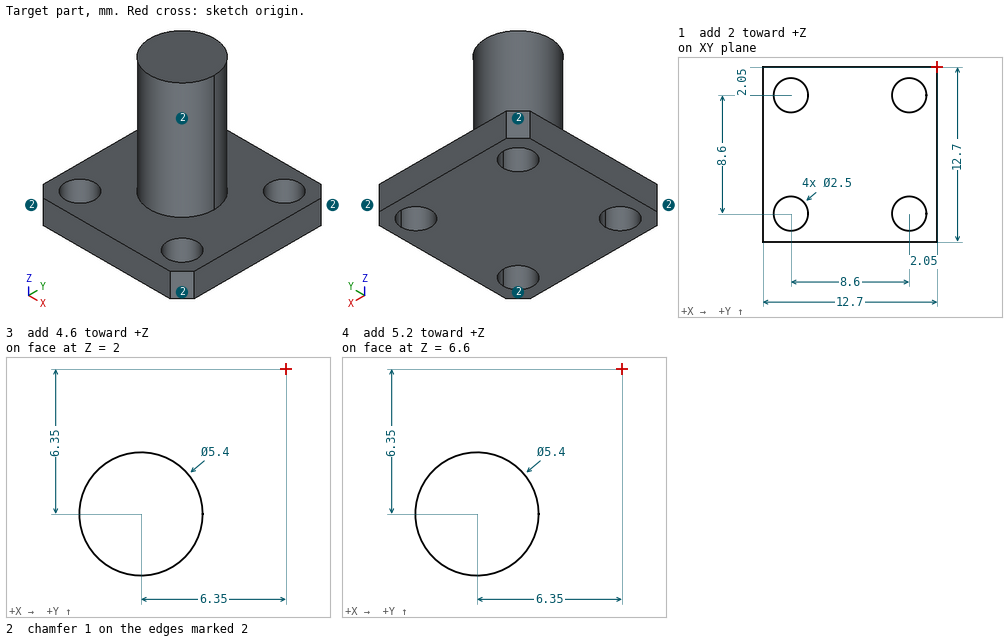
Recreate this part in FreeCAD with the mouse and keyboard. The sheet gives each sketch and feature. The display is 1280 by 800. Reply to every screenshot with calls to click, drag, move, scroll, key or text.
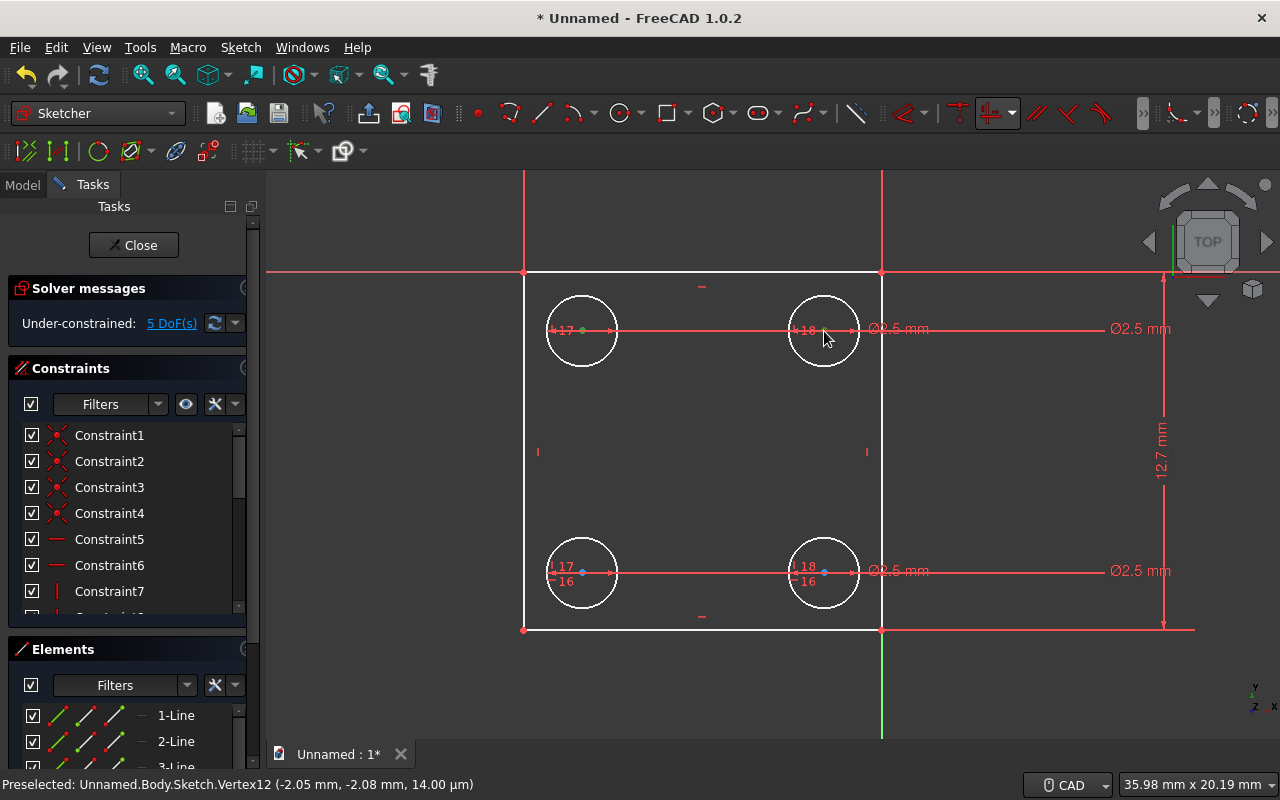
click(1014, 114)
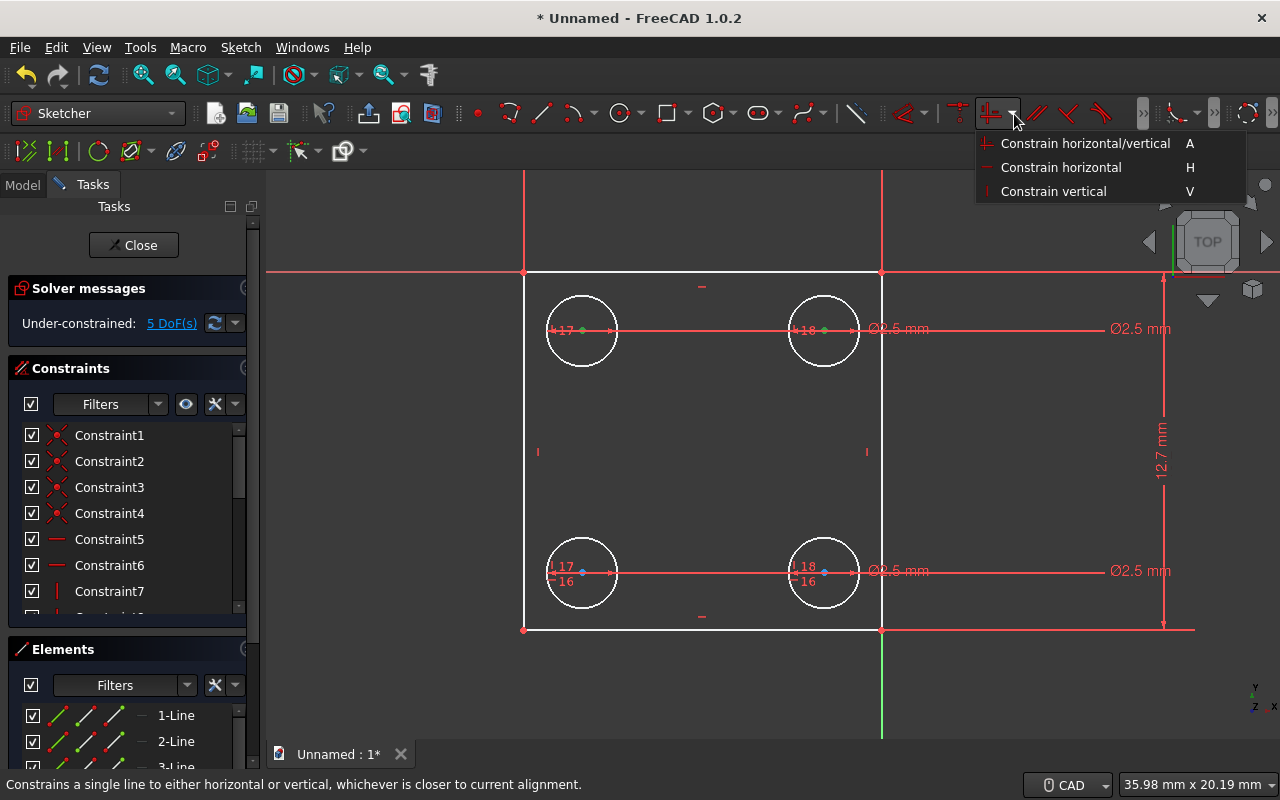
click(1111, 167)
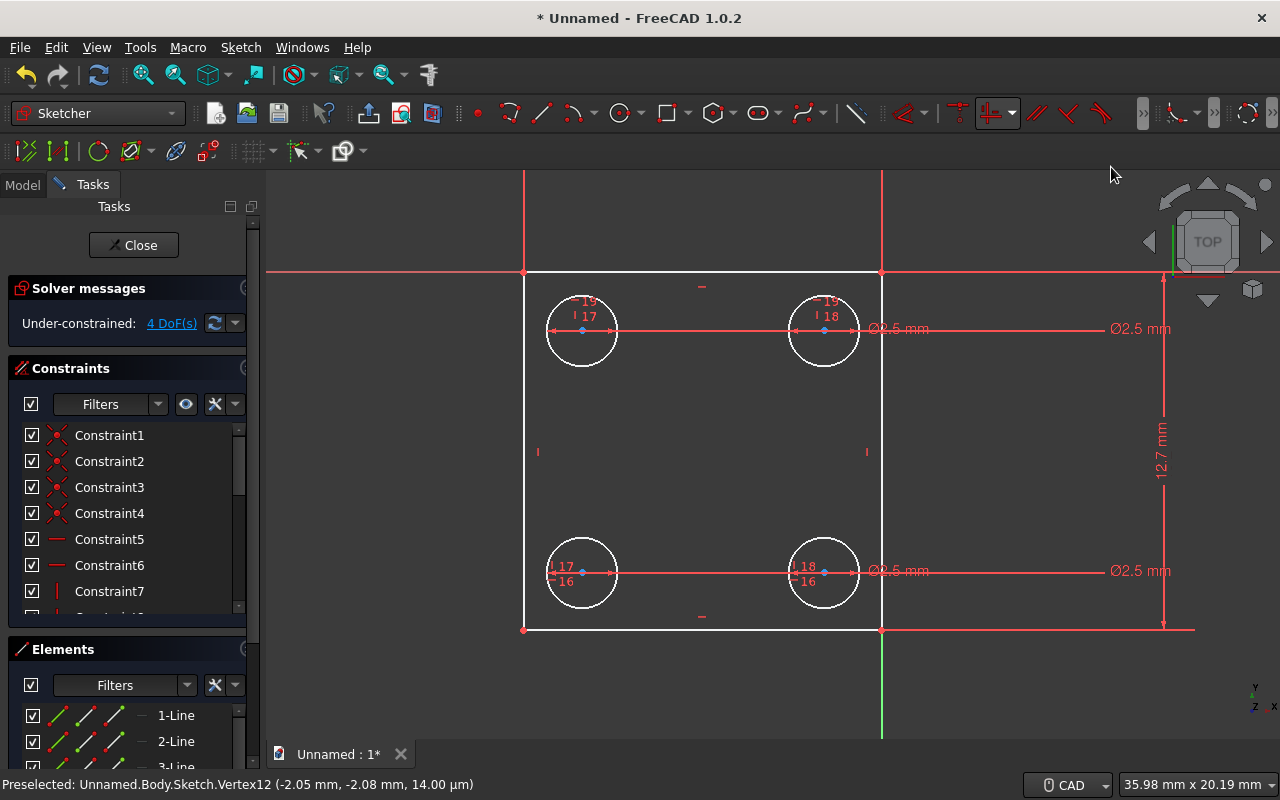
click(904, 114)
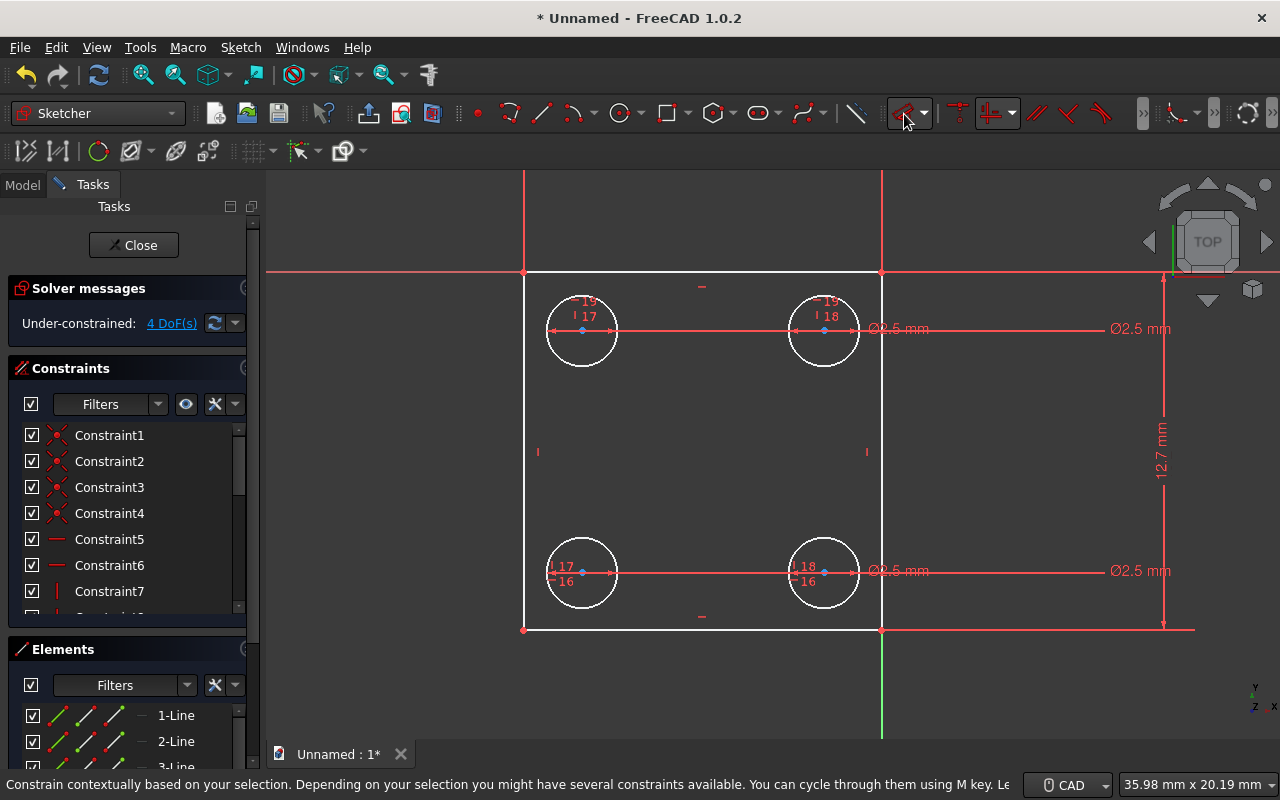
click(824, 573)
click(853, 238)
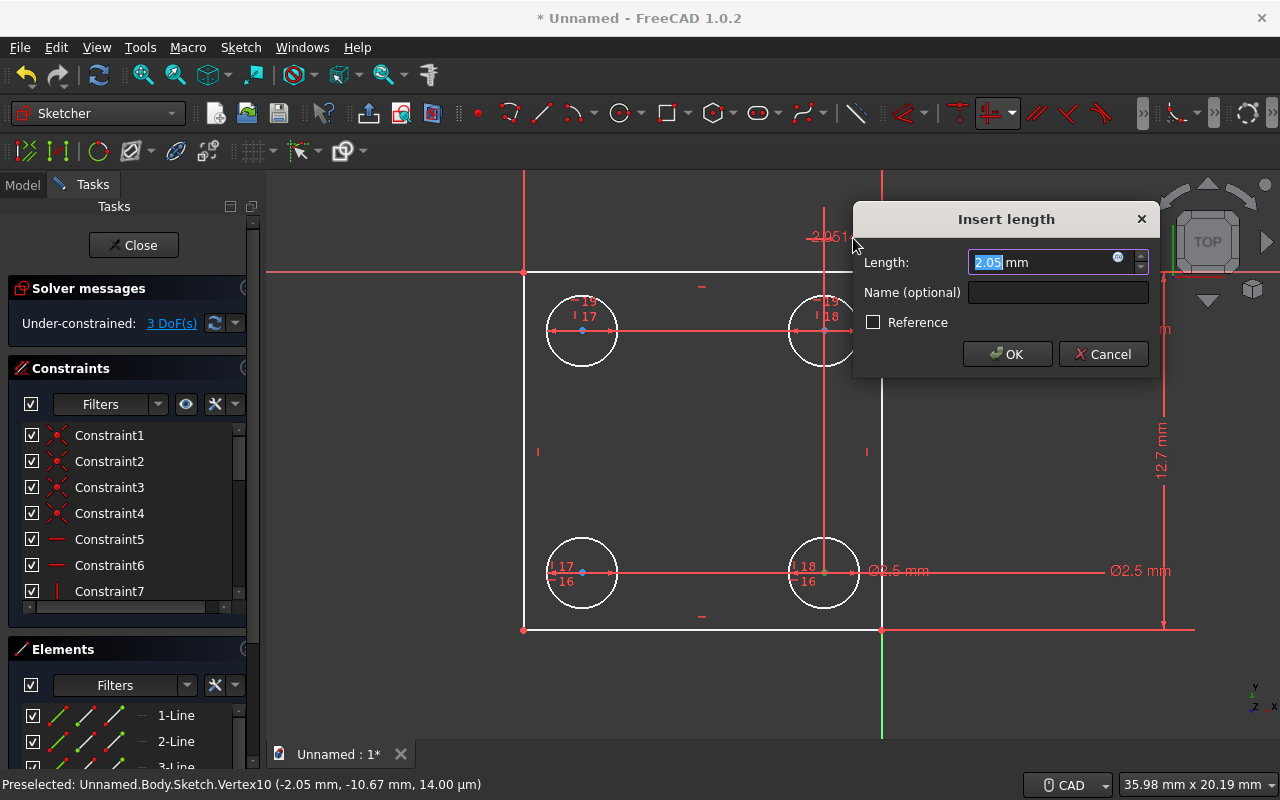
text(2.05)
key(Return)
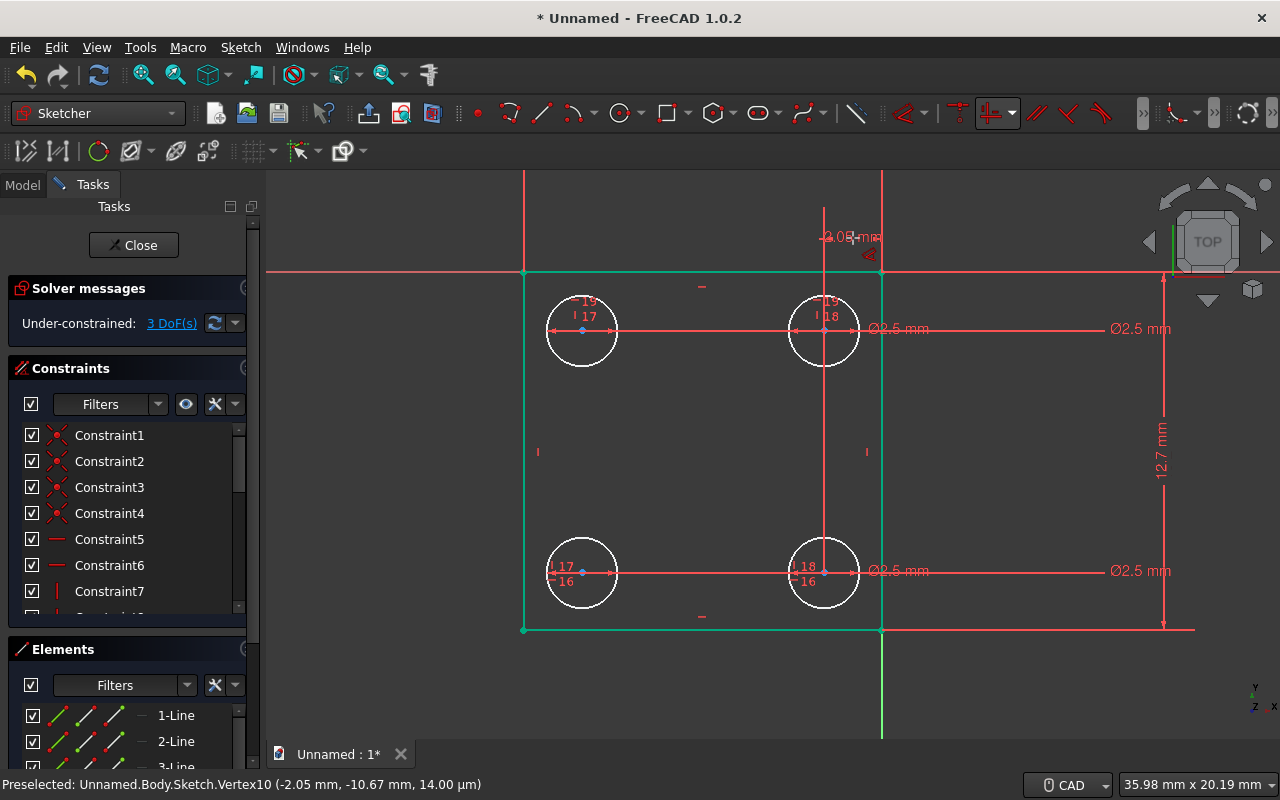
click(582, 331)
click(916, 302)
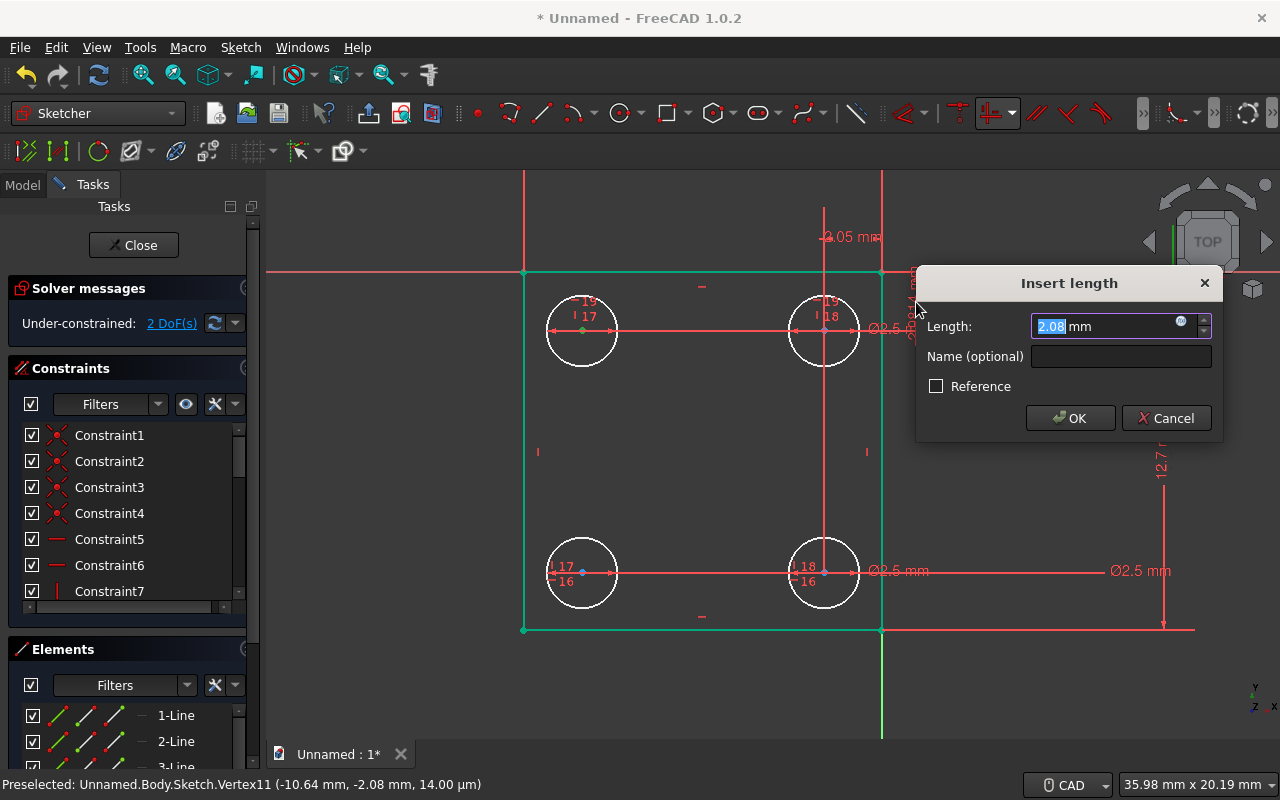
text(2.05)
key(Return)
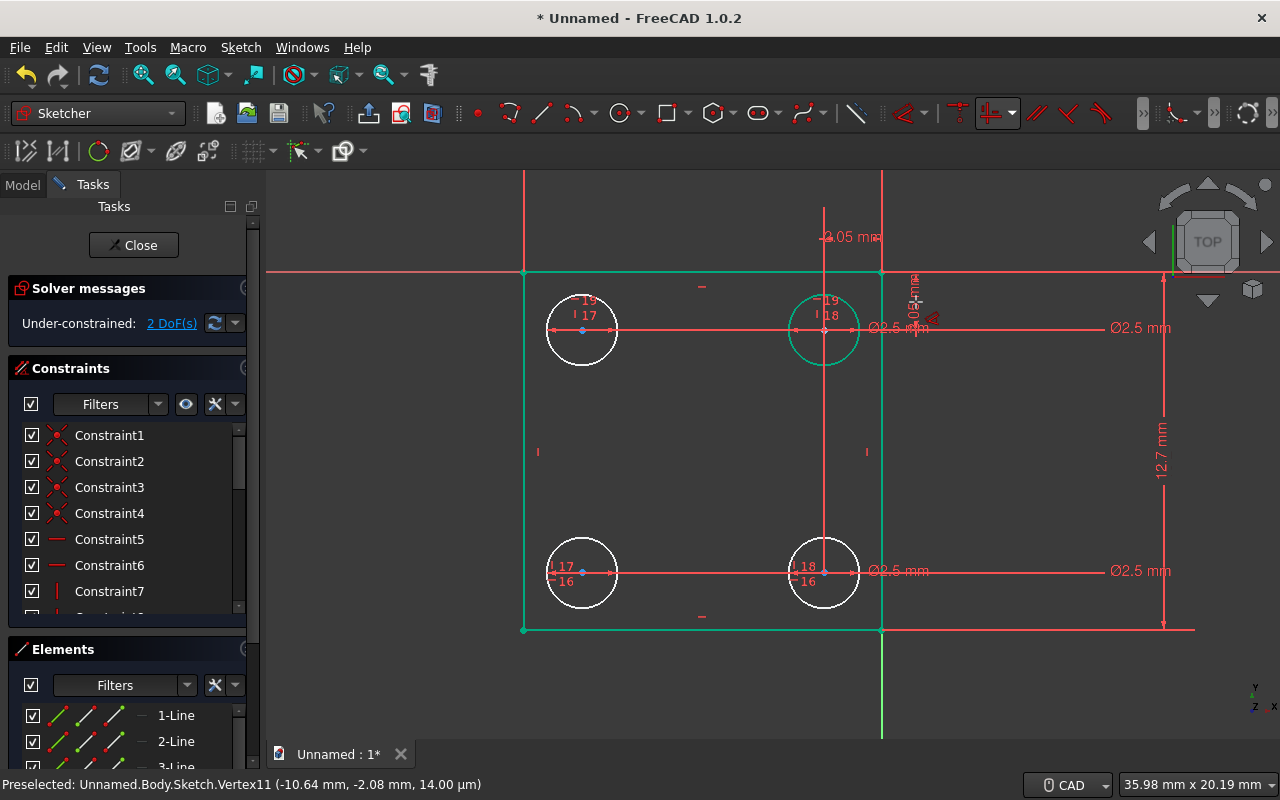
click(582, 573)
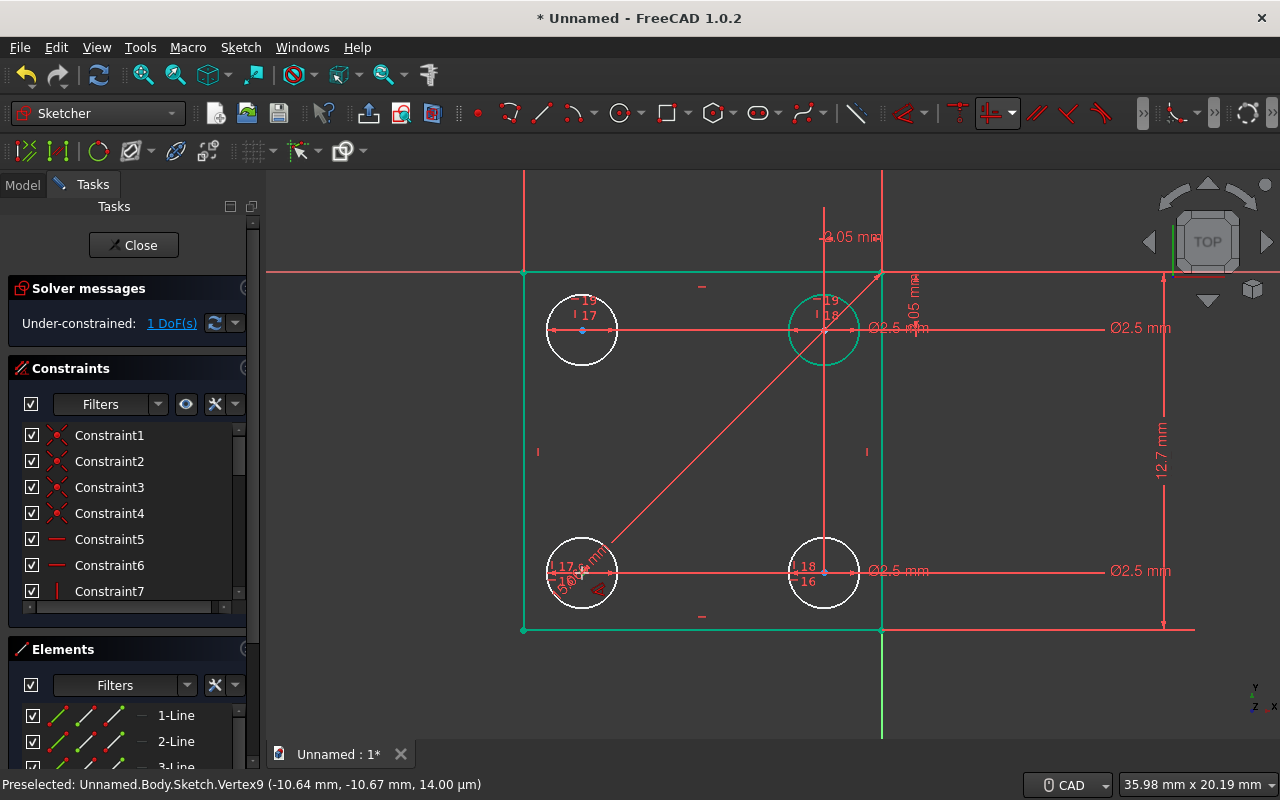
click(824, 573)
click(703, 607)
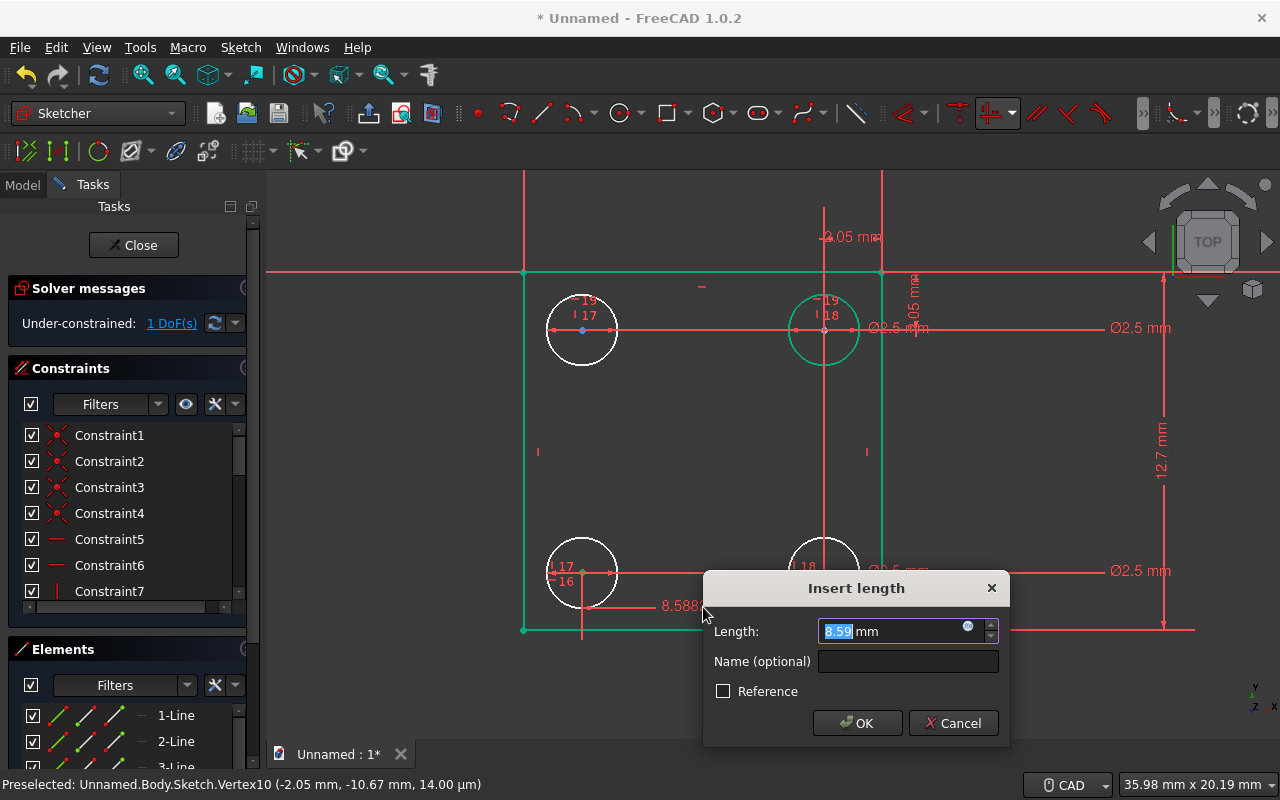
text(8.6)
key(Return)